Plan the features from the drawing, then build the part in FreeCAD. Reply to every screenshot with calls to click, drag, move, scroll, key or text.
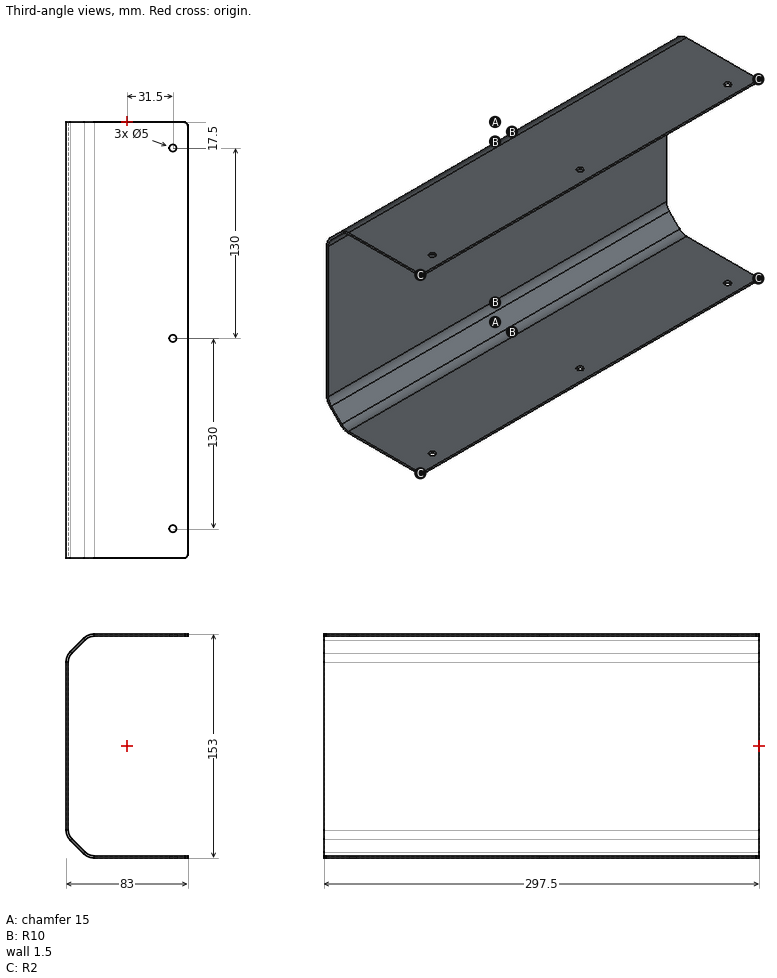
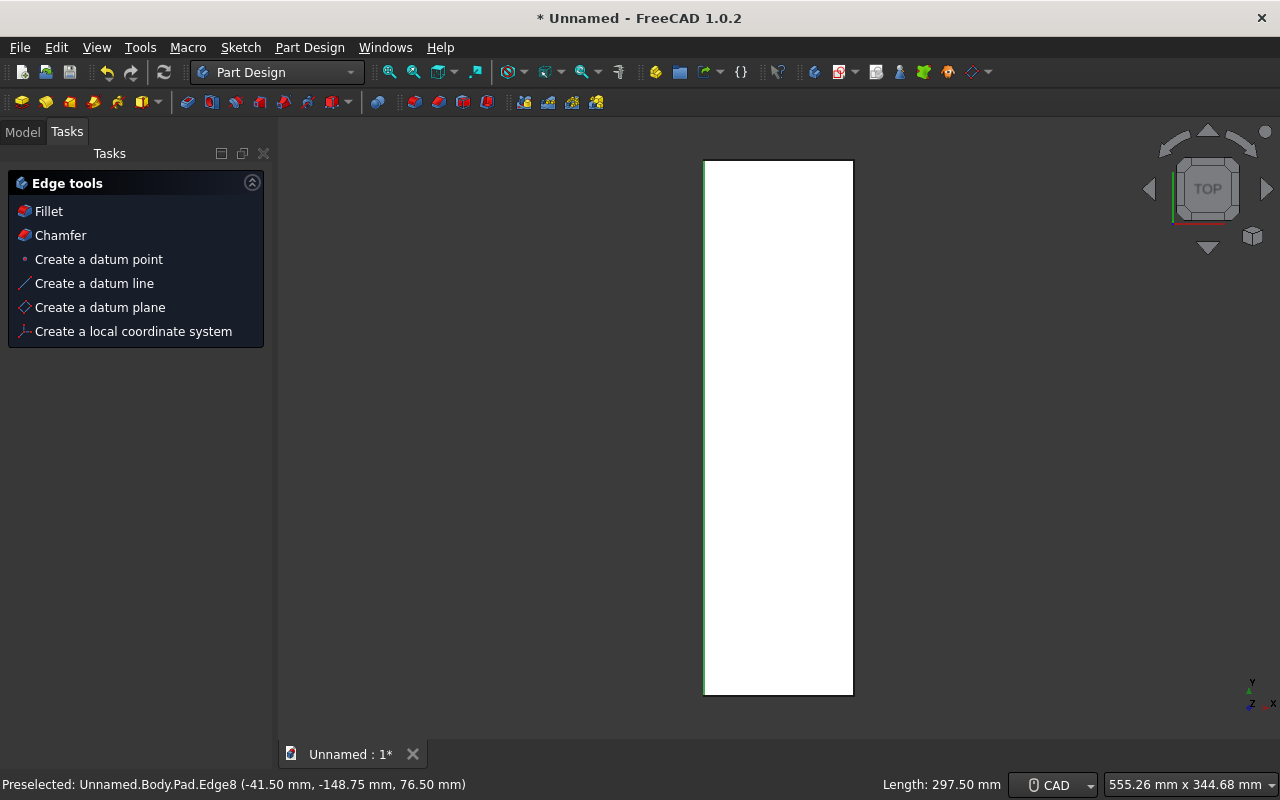
key(1)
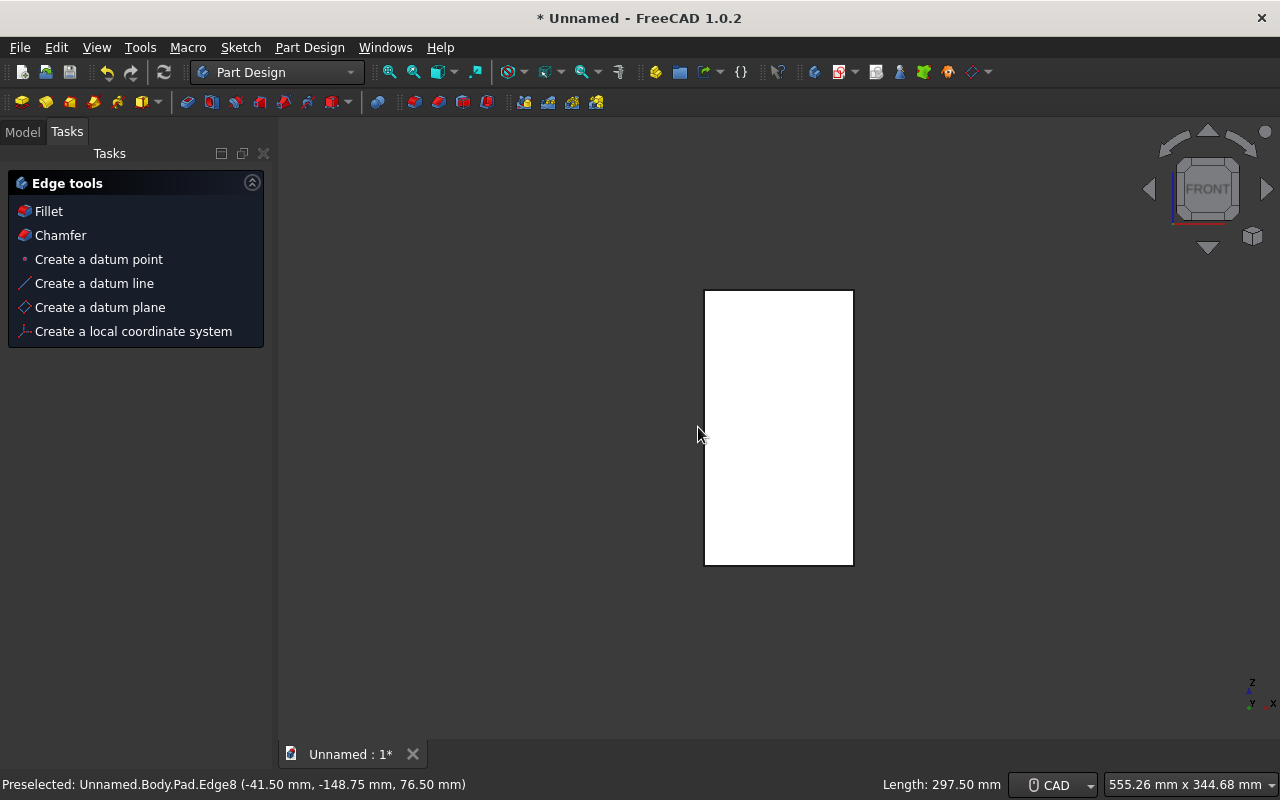
click(390, 72)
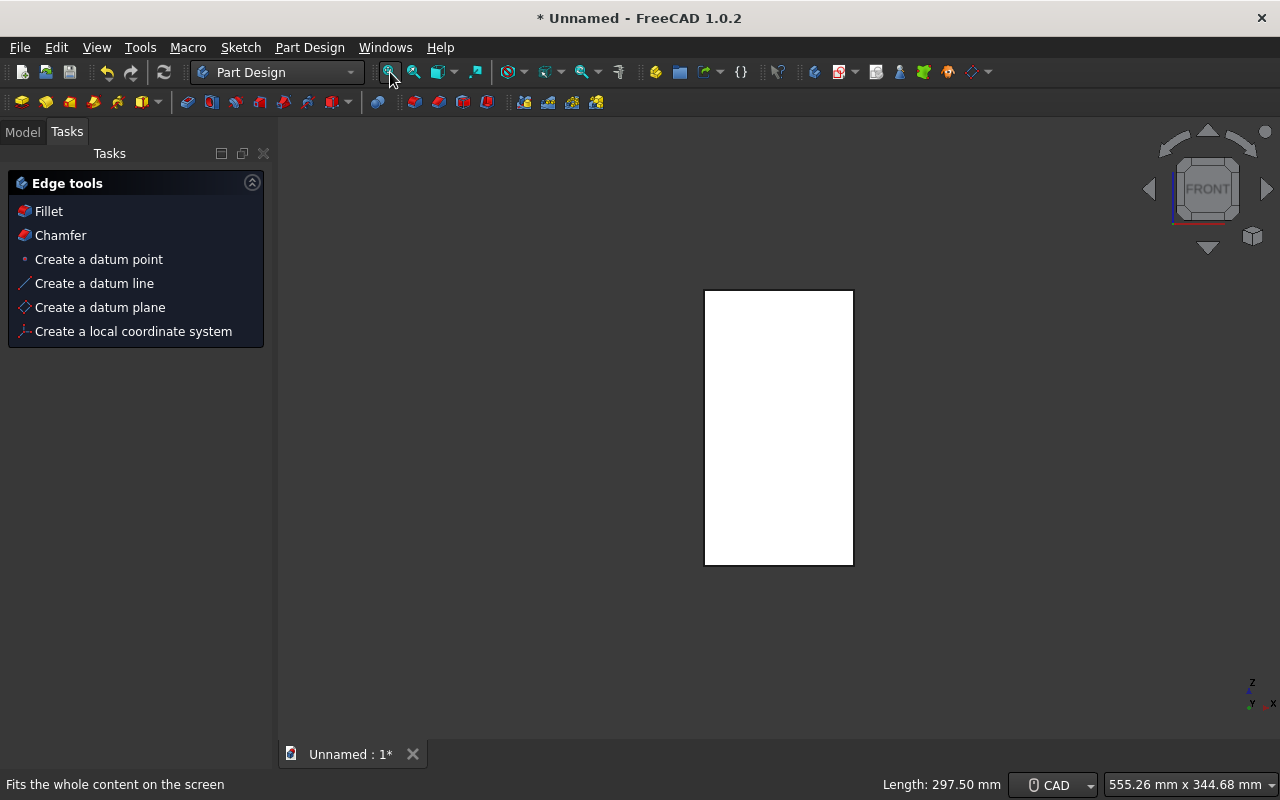
key(3)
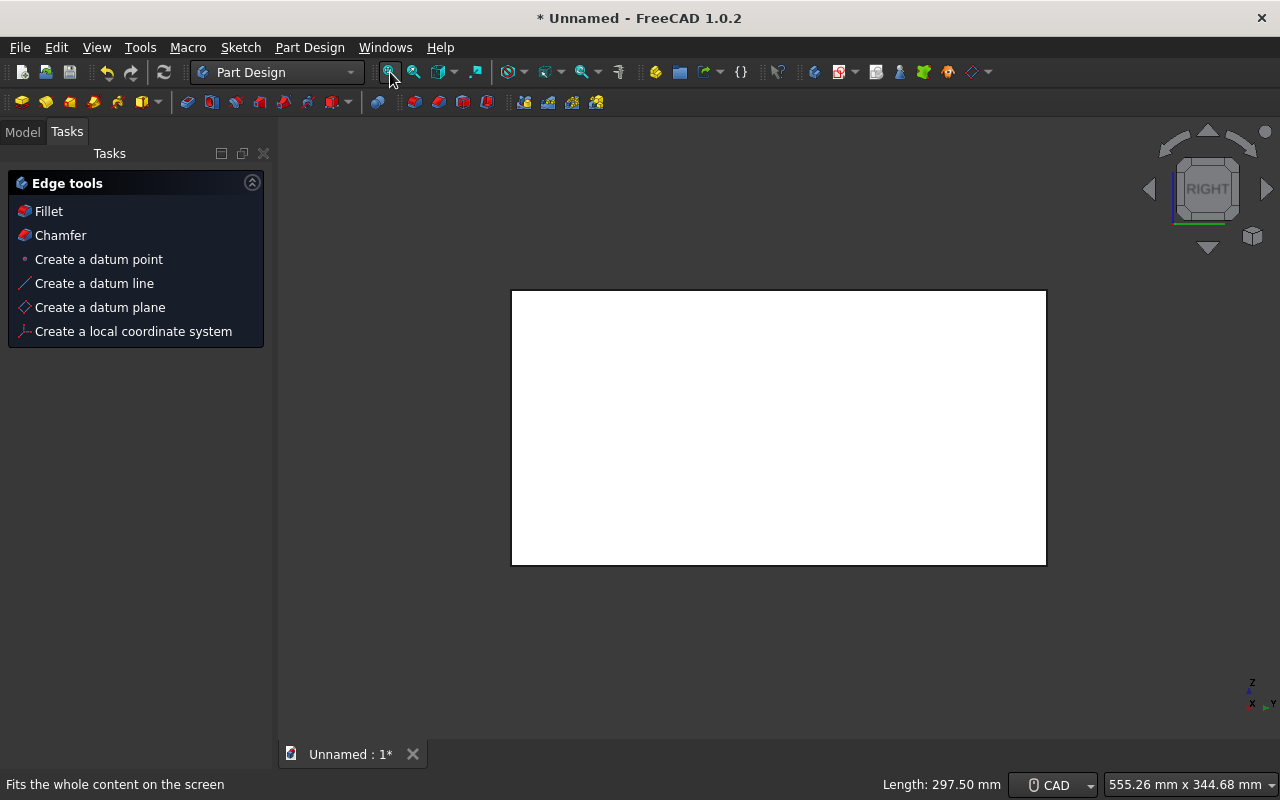
key(5)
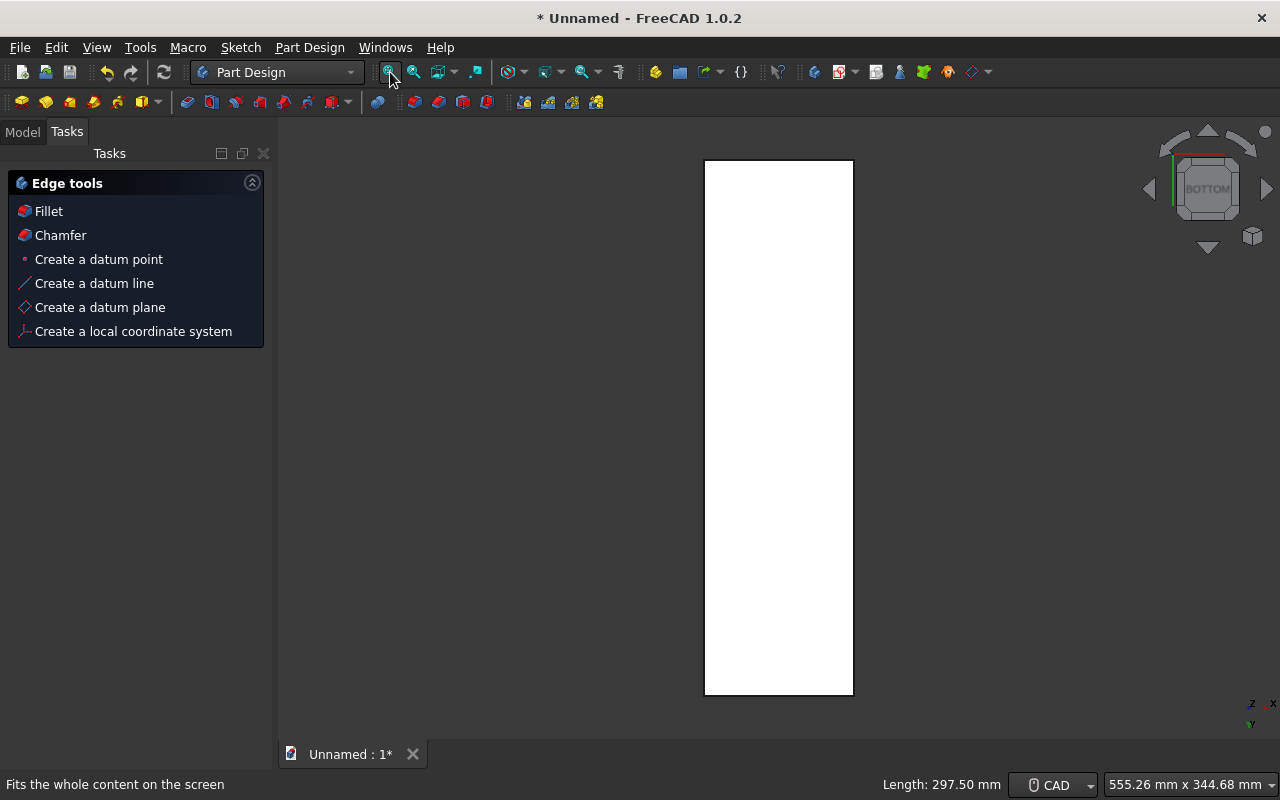
click(704, 427, ctrl)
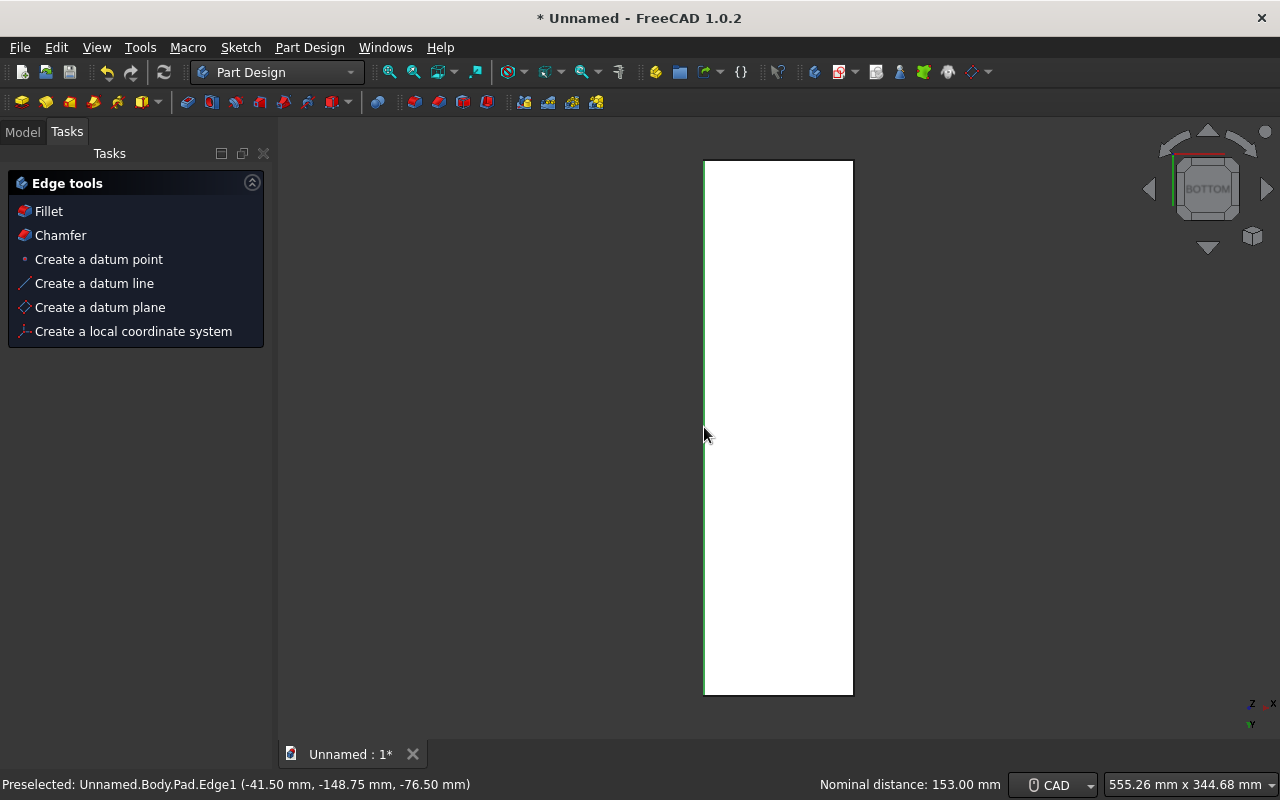
click(440, 102)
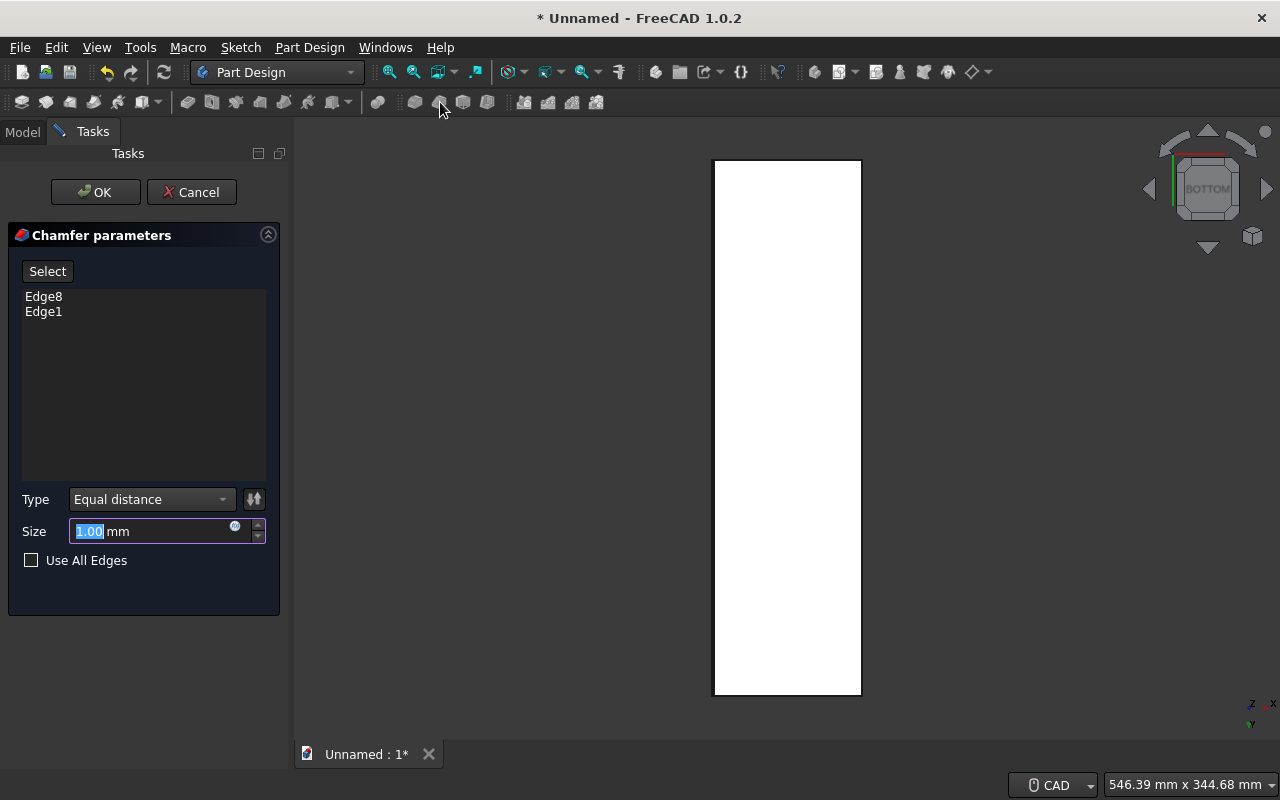
text(15)
key(Tab)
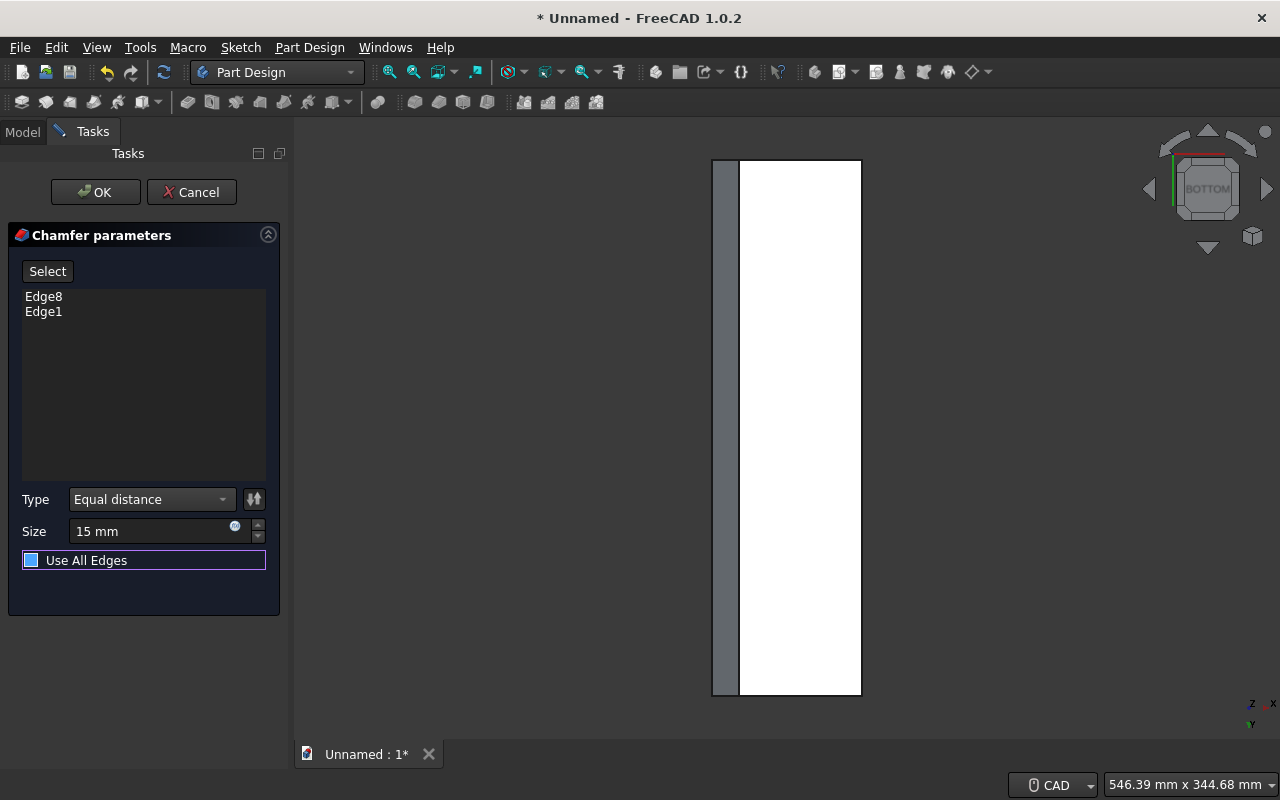
click(96, 192)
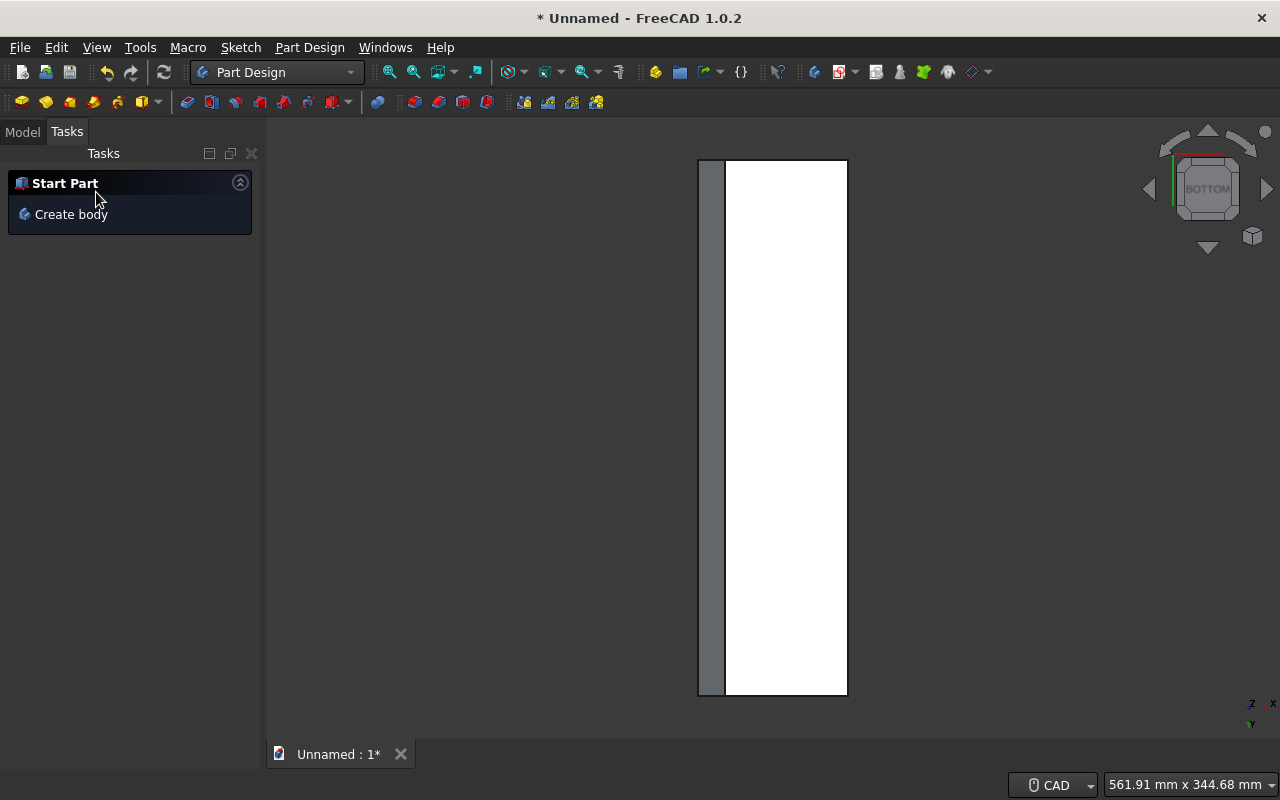
click(725, 427)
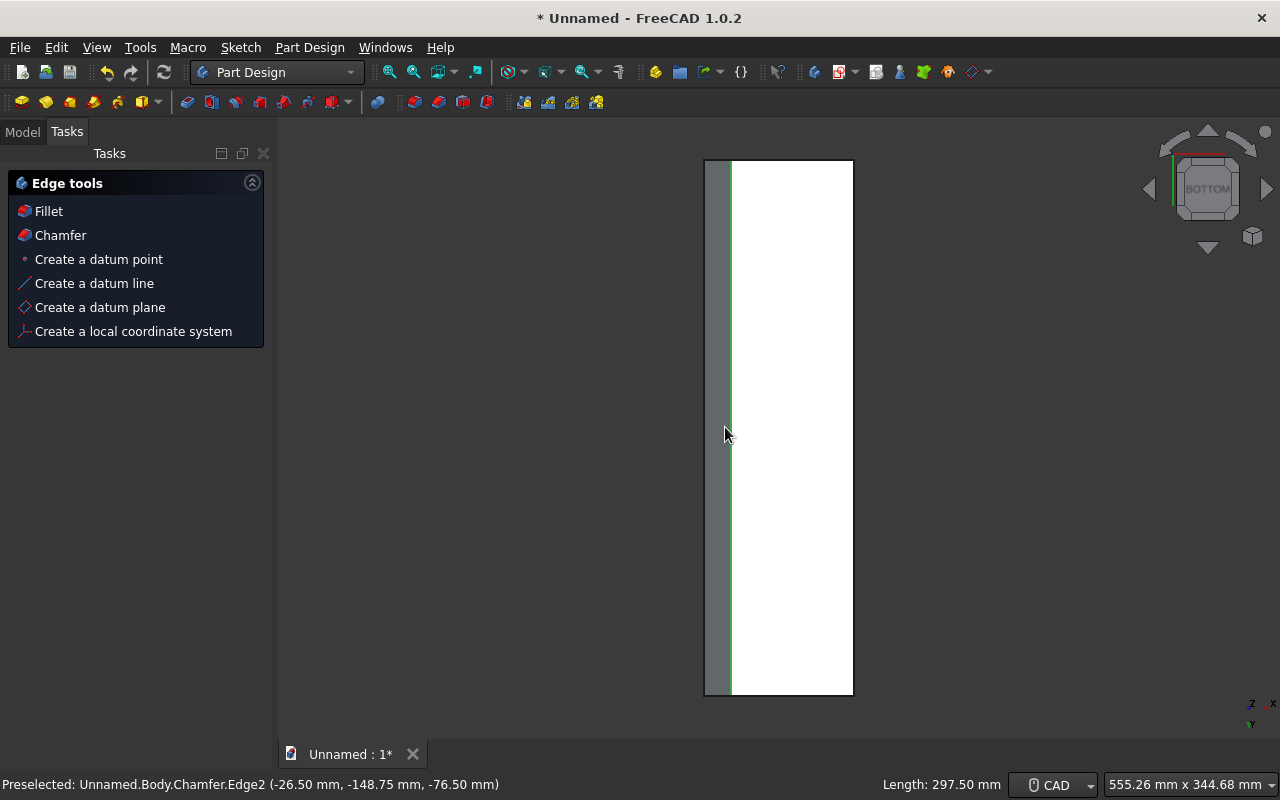
key(0)